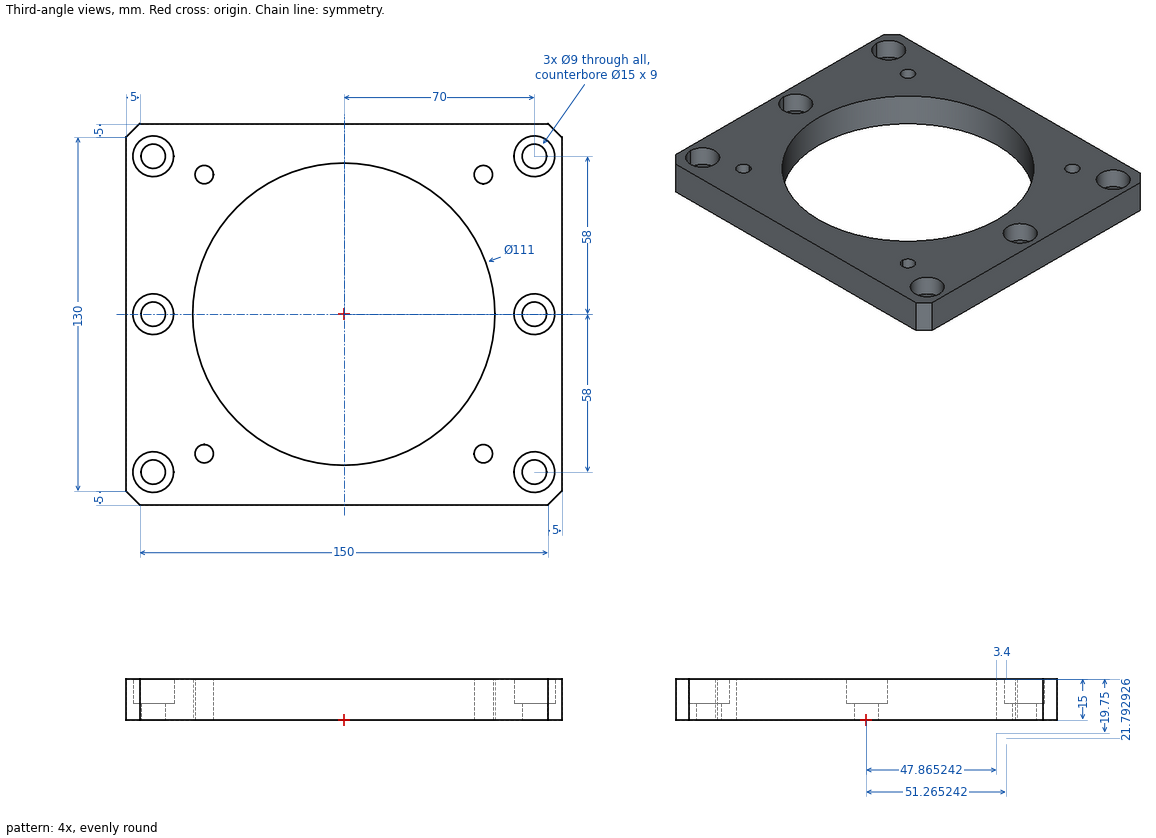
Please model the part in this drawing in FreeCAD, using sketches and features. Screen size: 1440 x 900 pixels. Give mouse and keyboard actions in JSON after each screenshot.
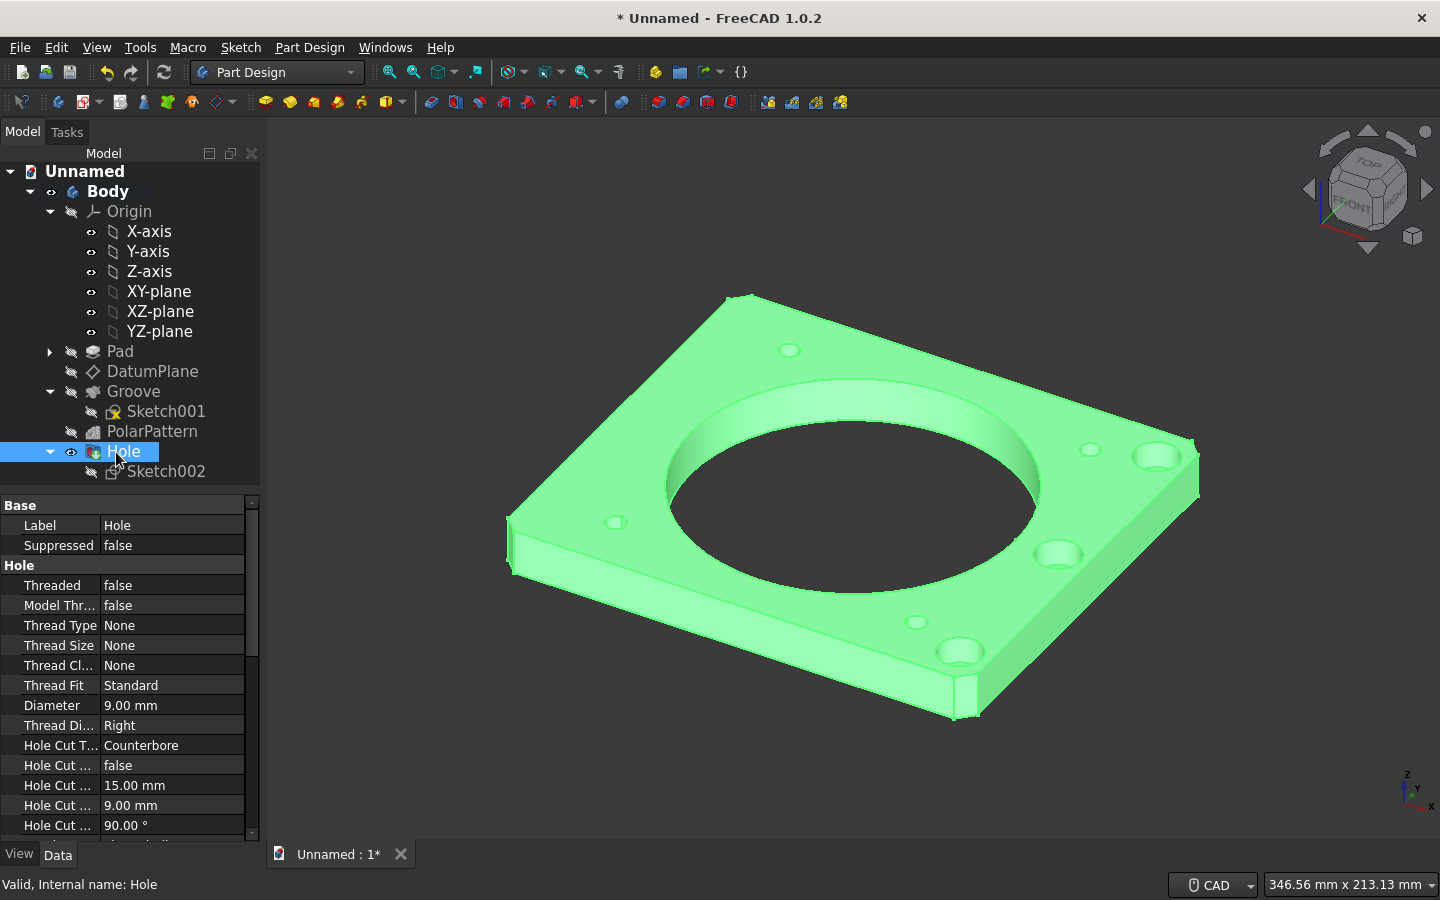
{"action": "left_click", "coordinate": [768, 102]}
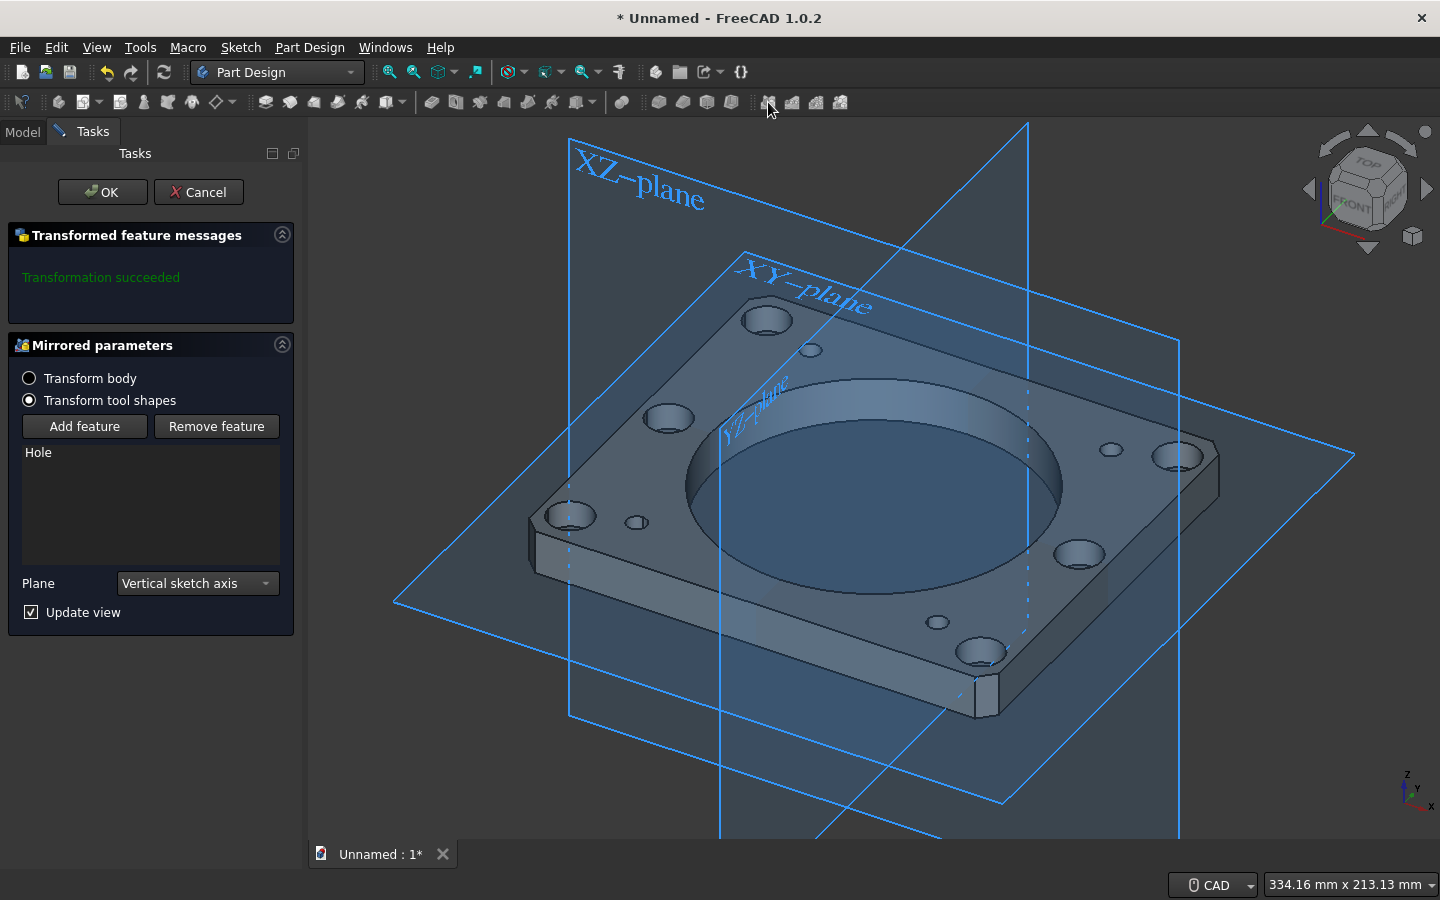
{"action": "left_click", "coordinate": [198, 584]}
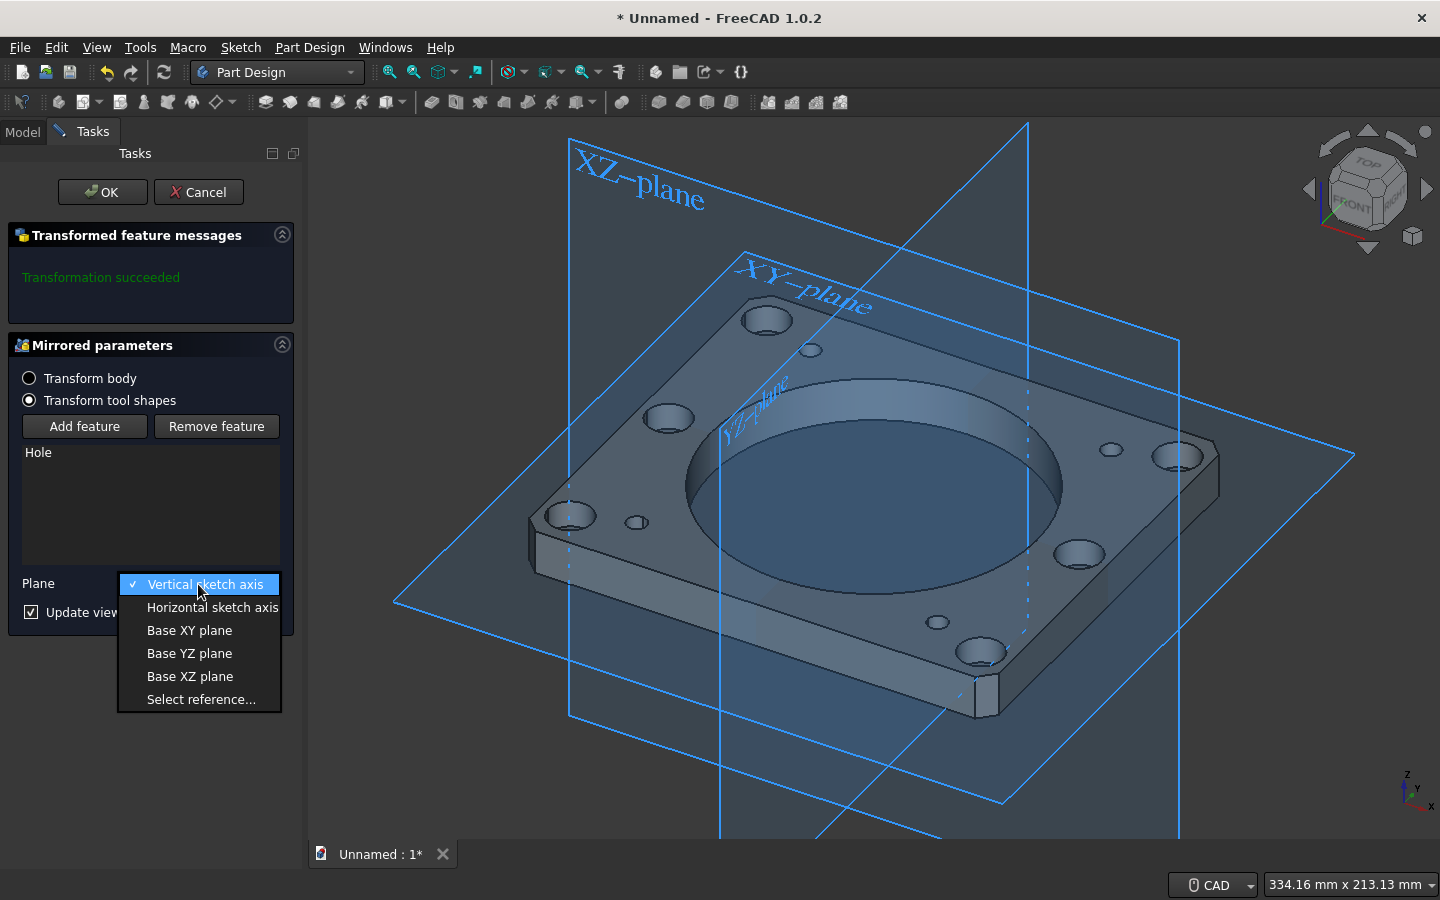
{"action": "left_click", "coordinate": [198, 654]}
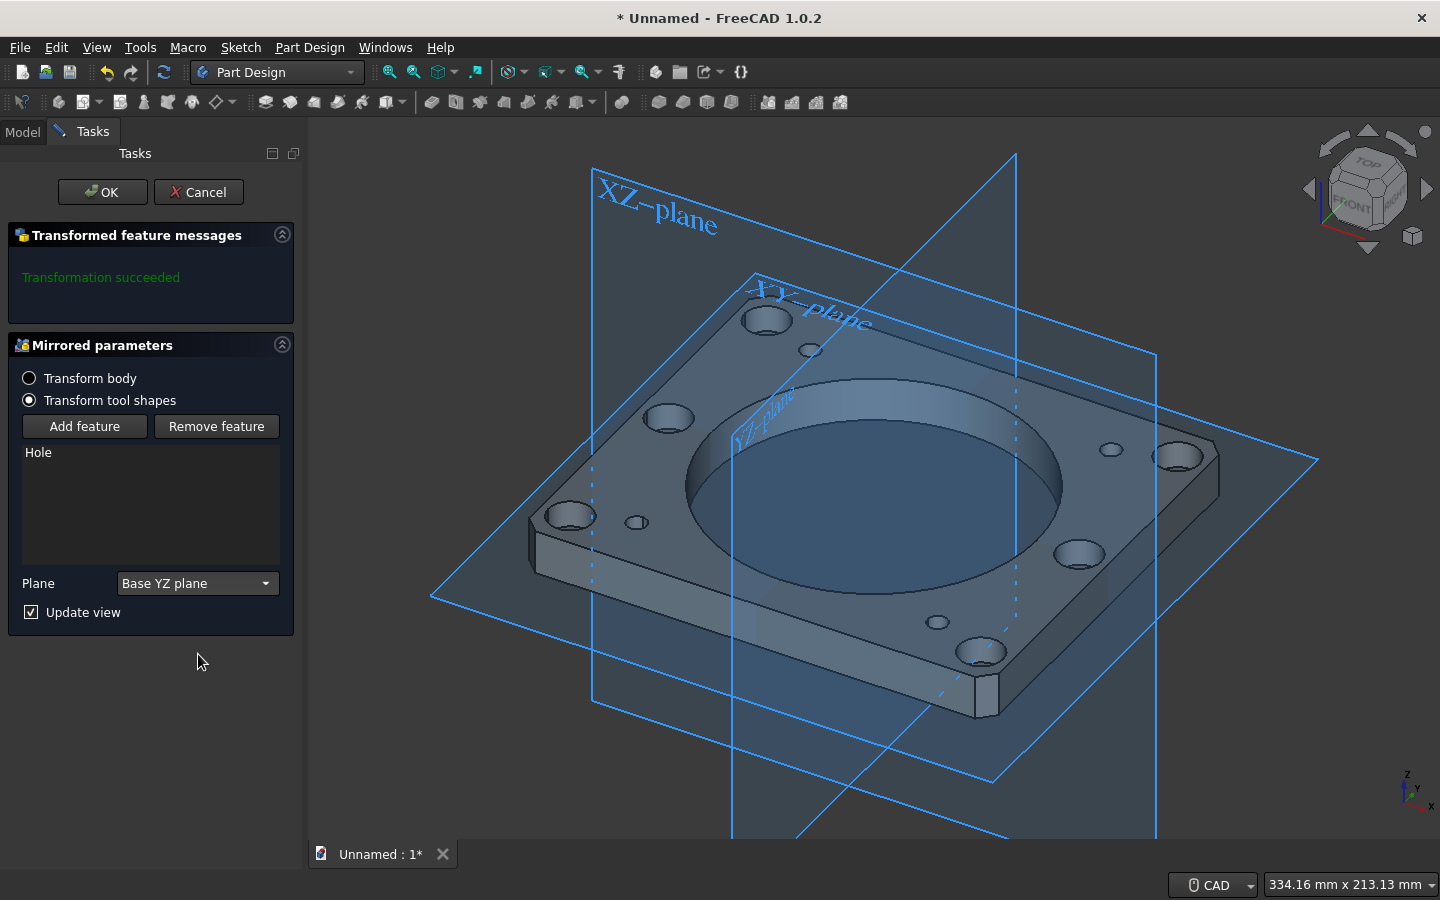
{"action": "left_click", "coordinate": [103, 192]}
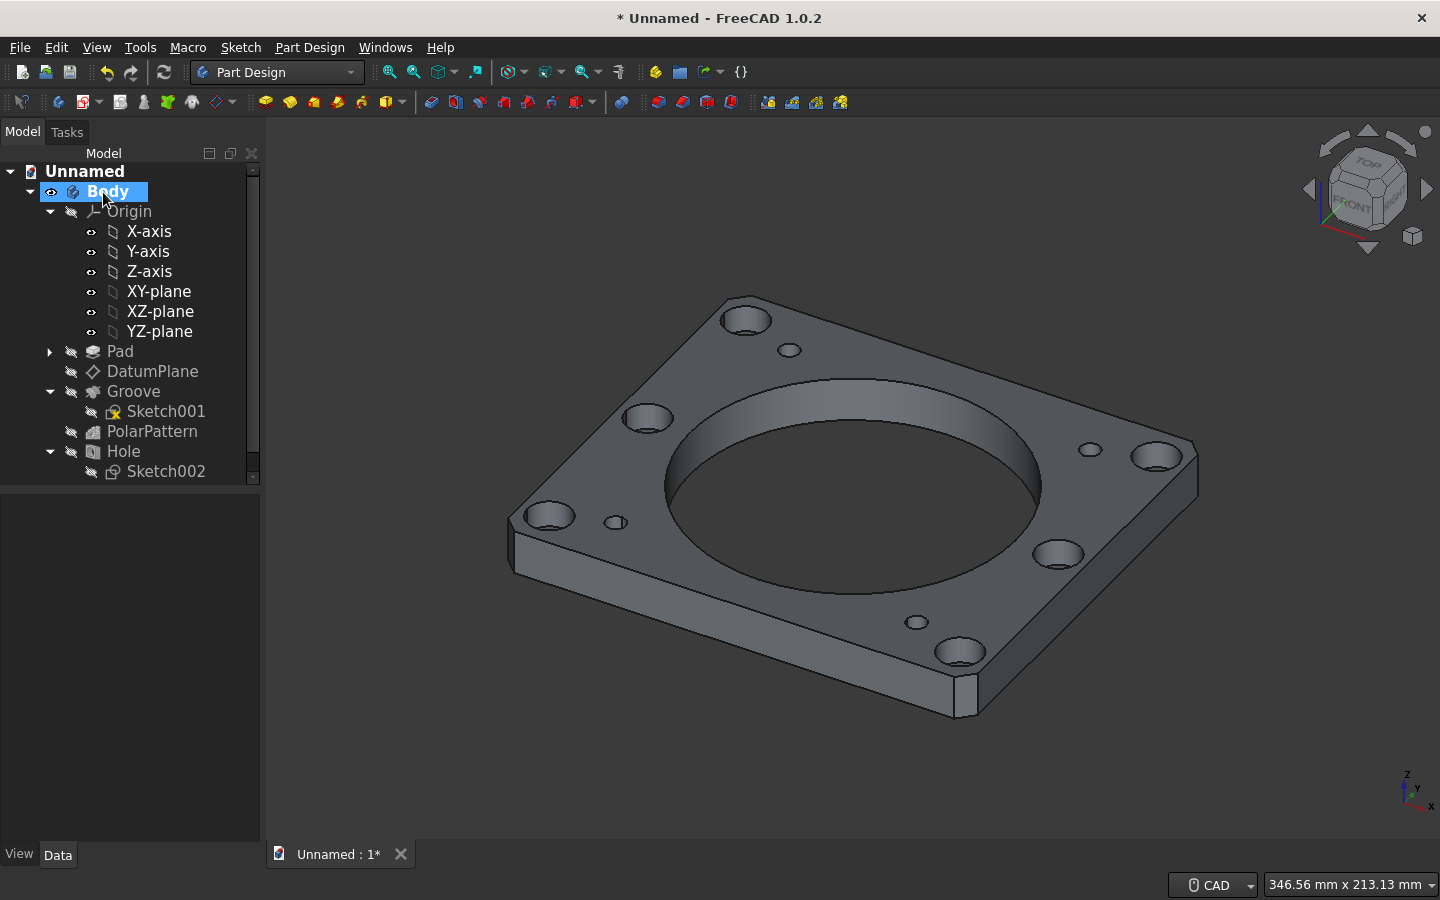
{"action": "key", "text": "0"}